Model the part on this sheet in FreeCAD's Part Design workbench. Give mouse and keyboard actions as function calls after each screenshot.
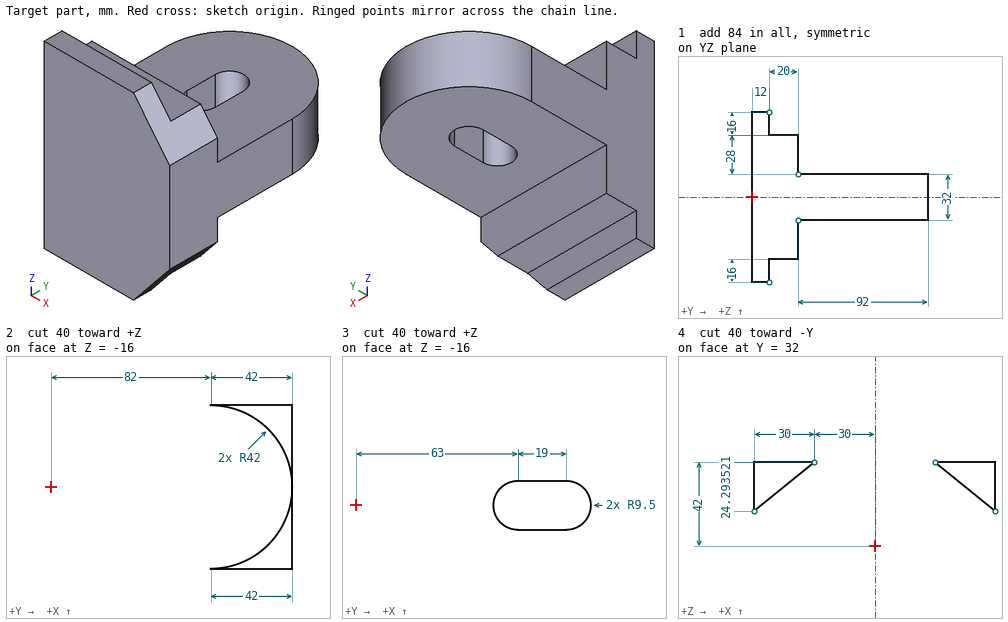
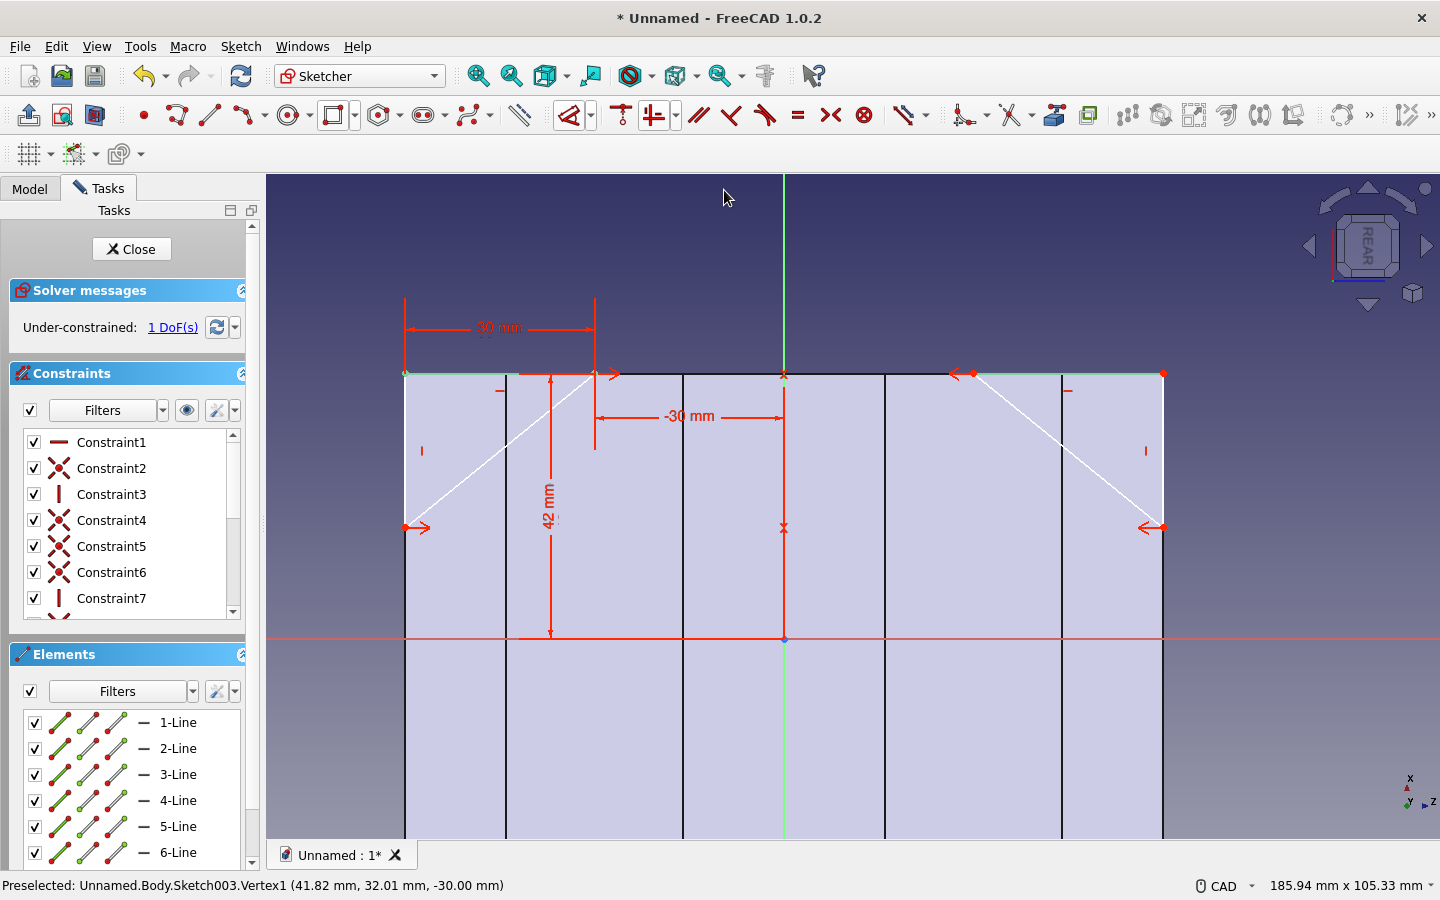
click(405, 420)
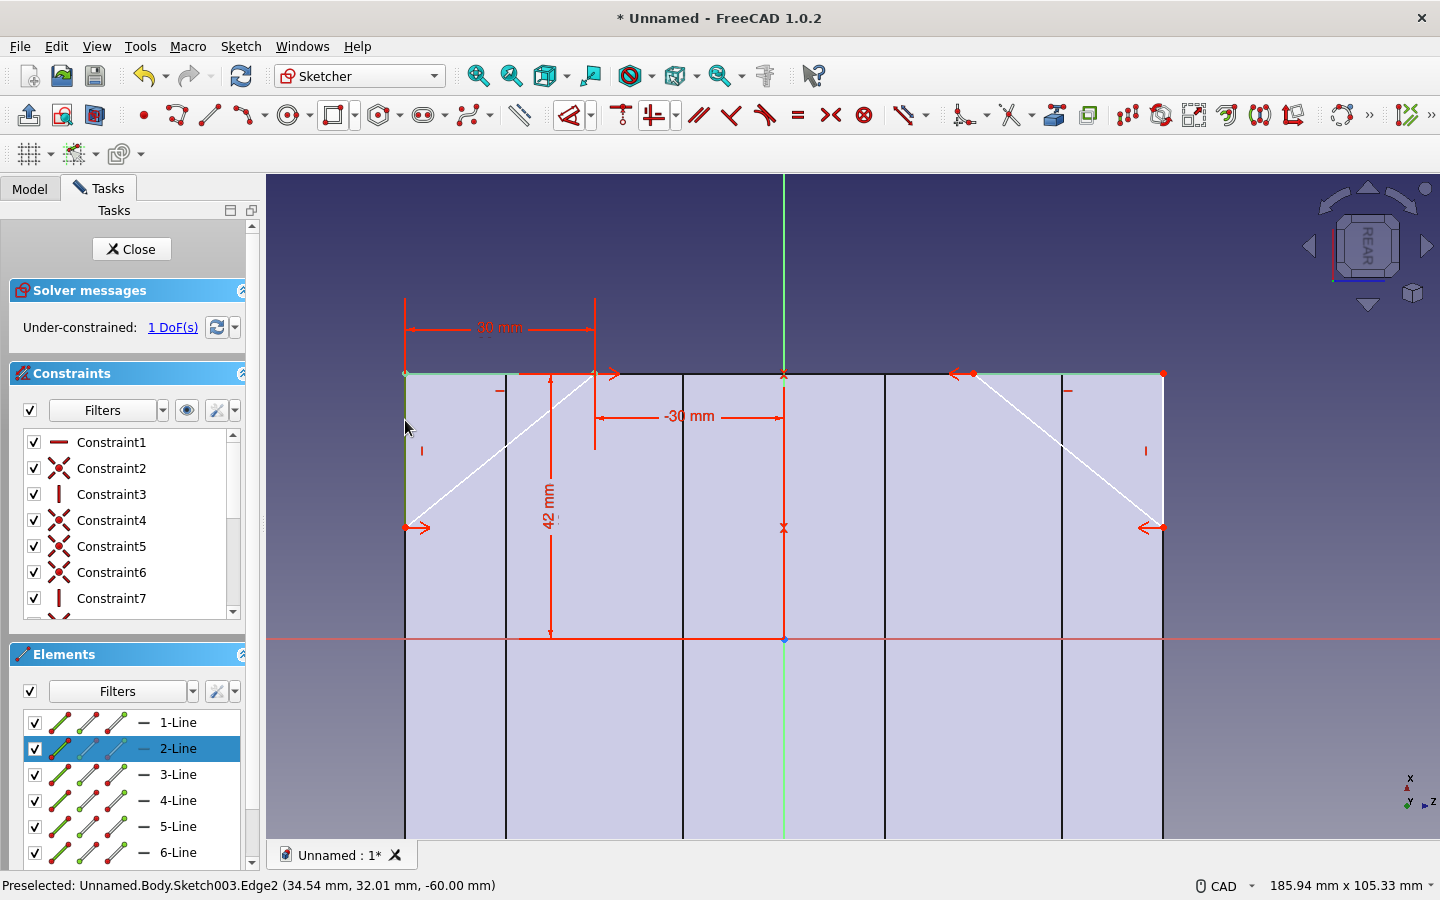
key(i)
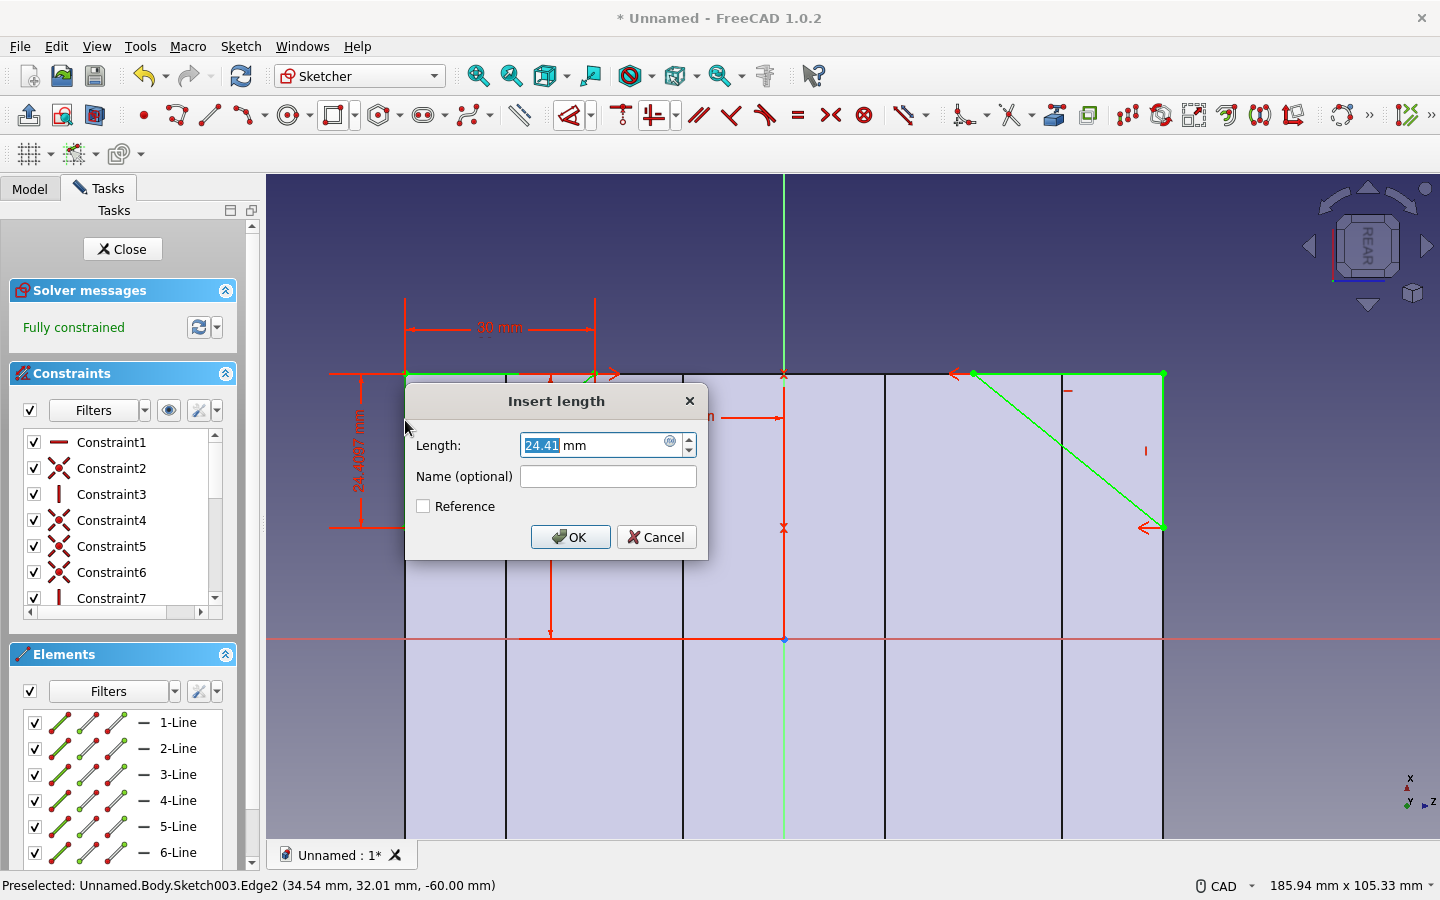
text(24.293521)
key(Return)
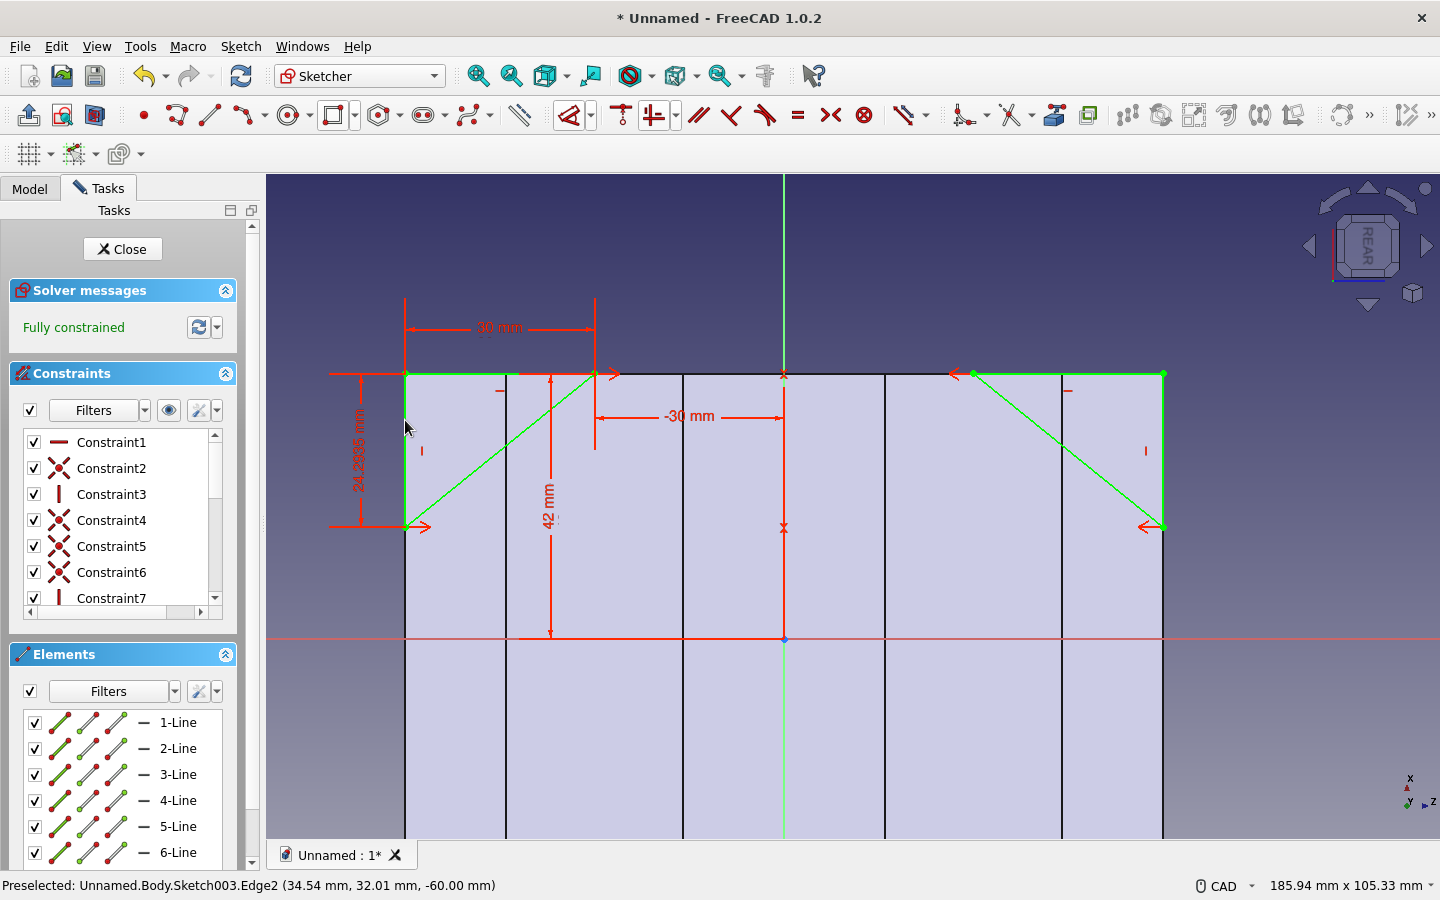
click(123, 249)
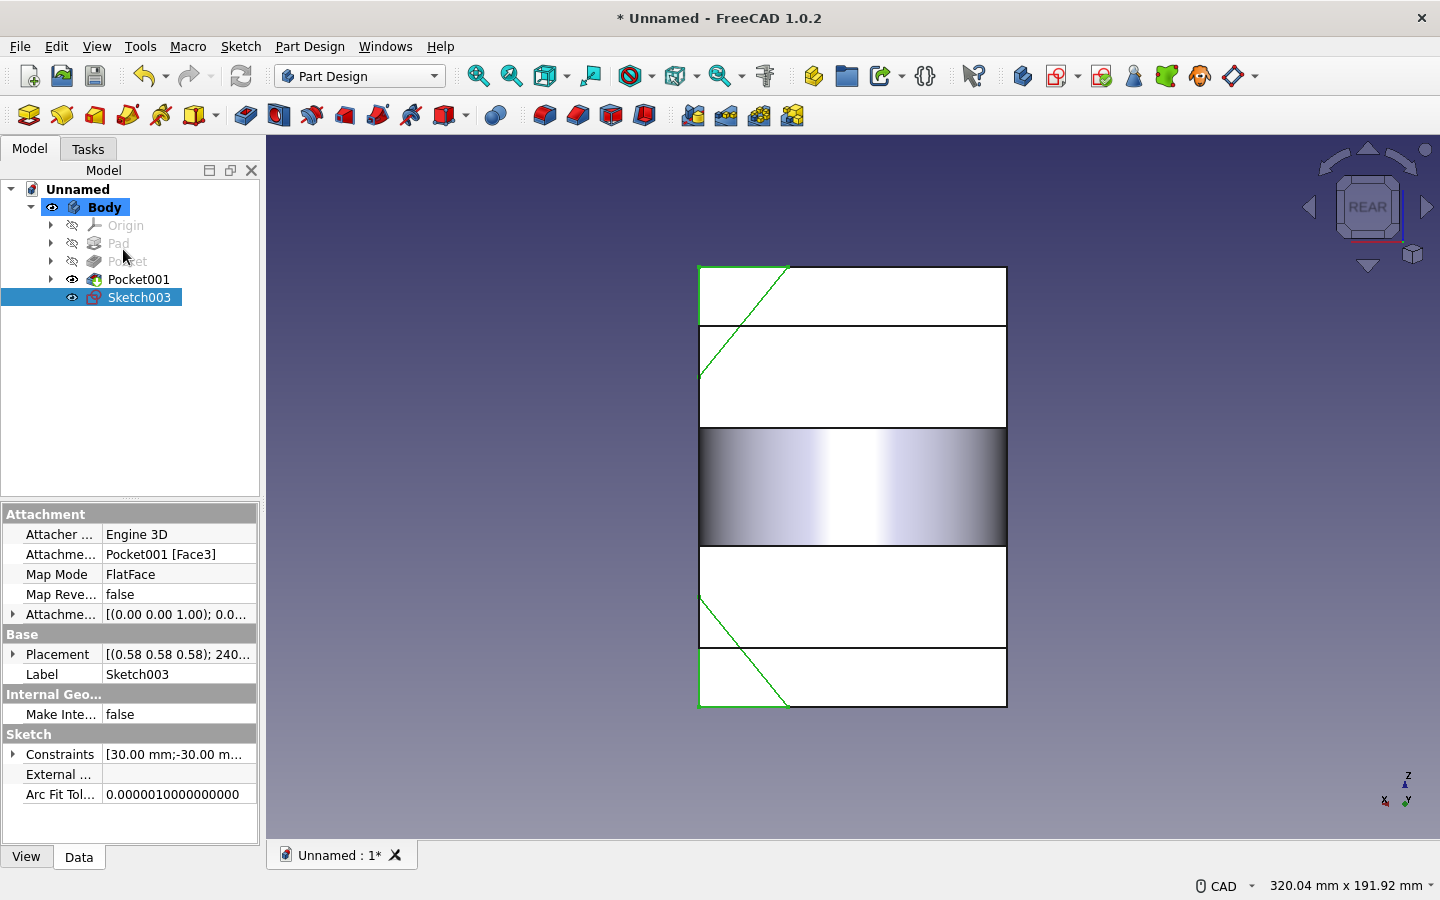
click(246, 116)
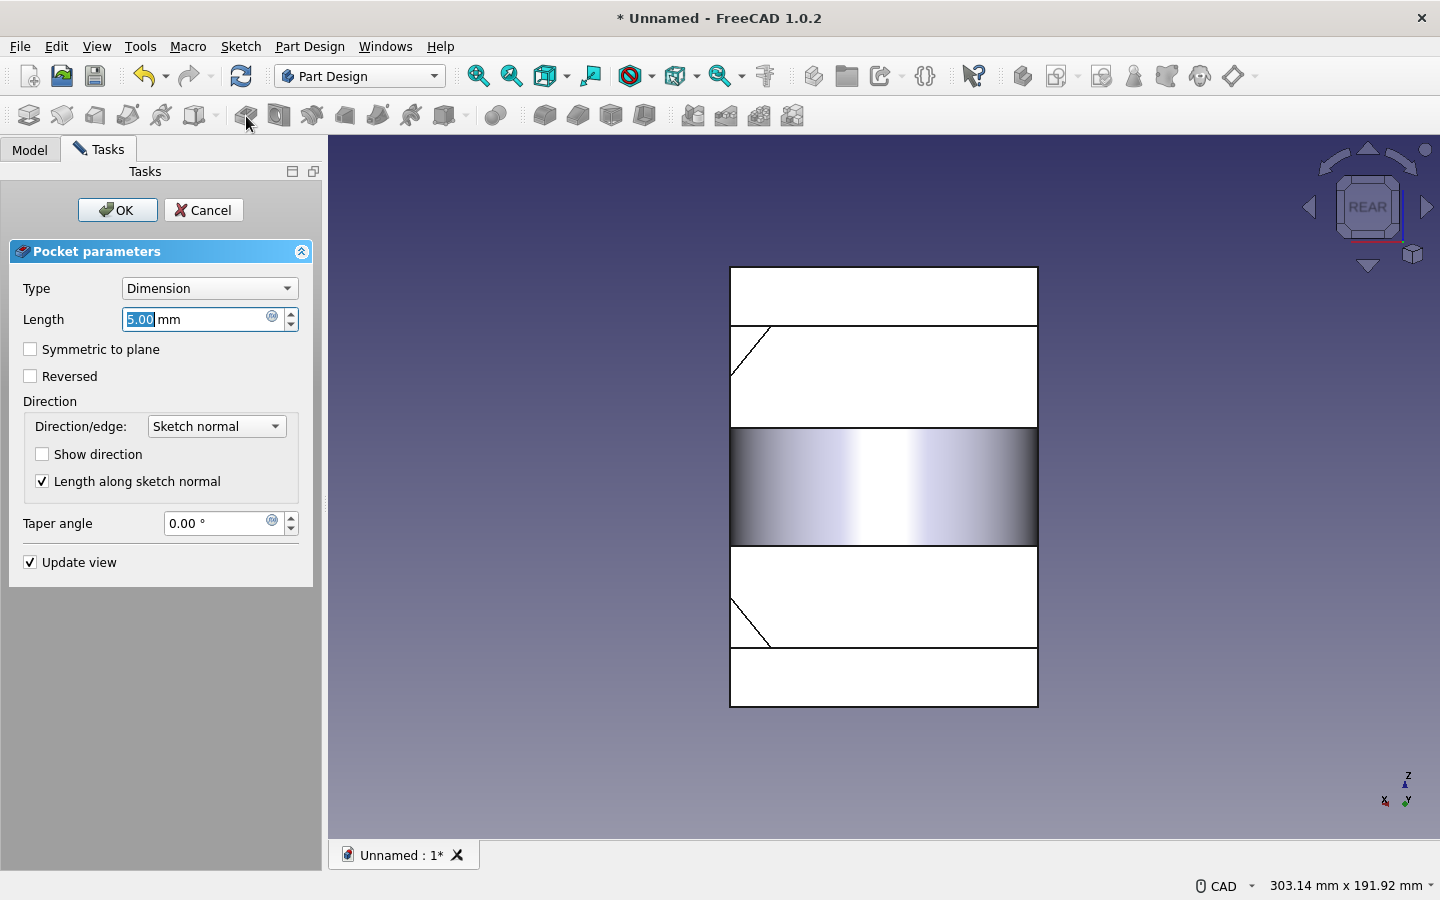
text(40)
key(Tab)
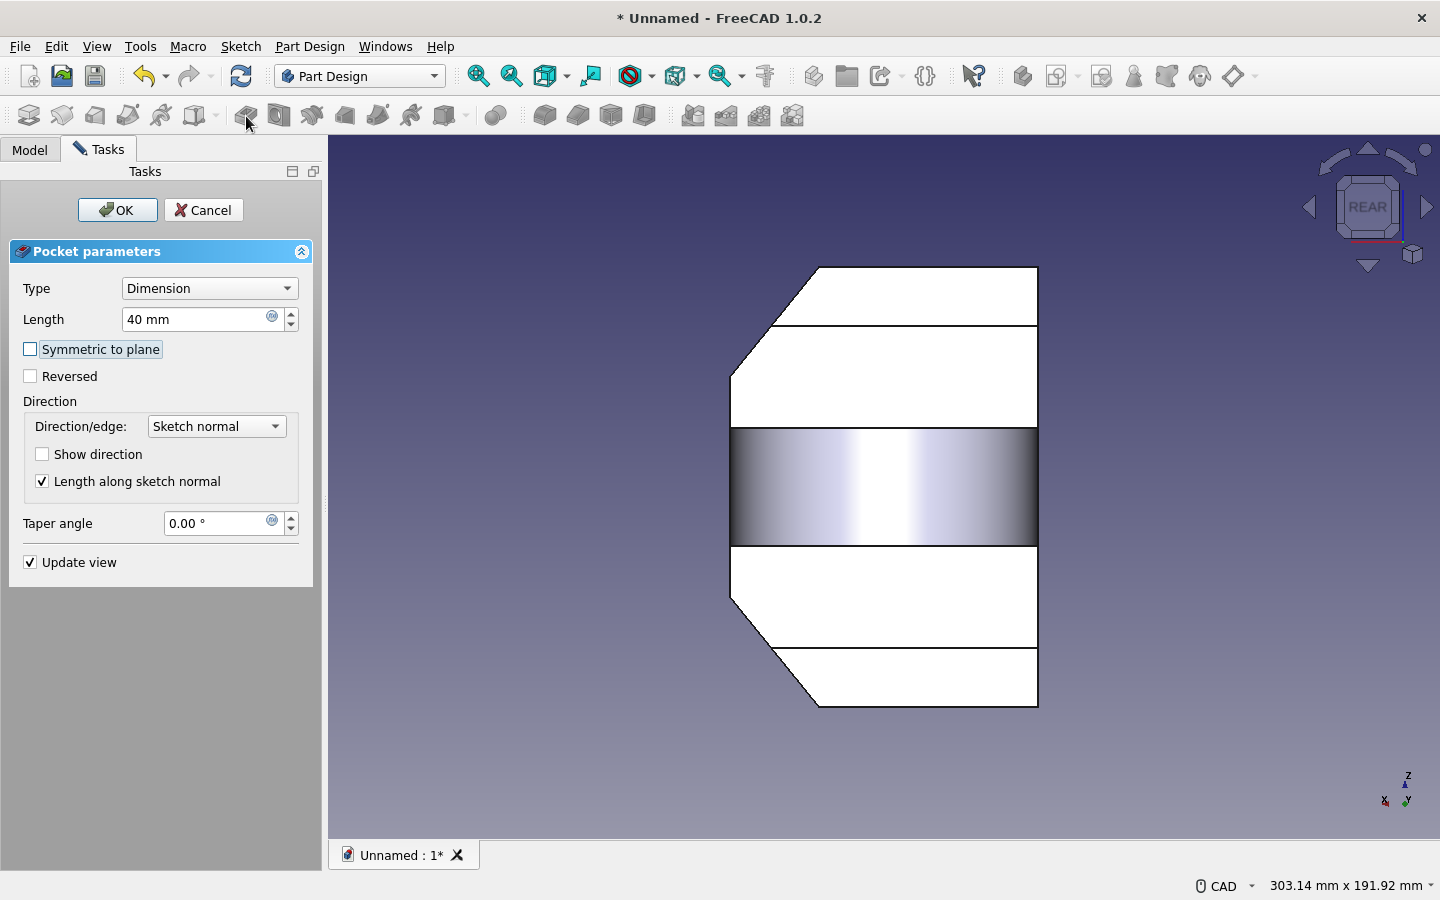
click(118, 210)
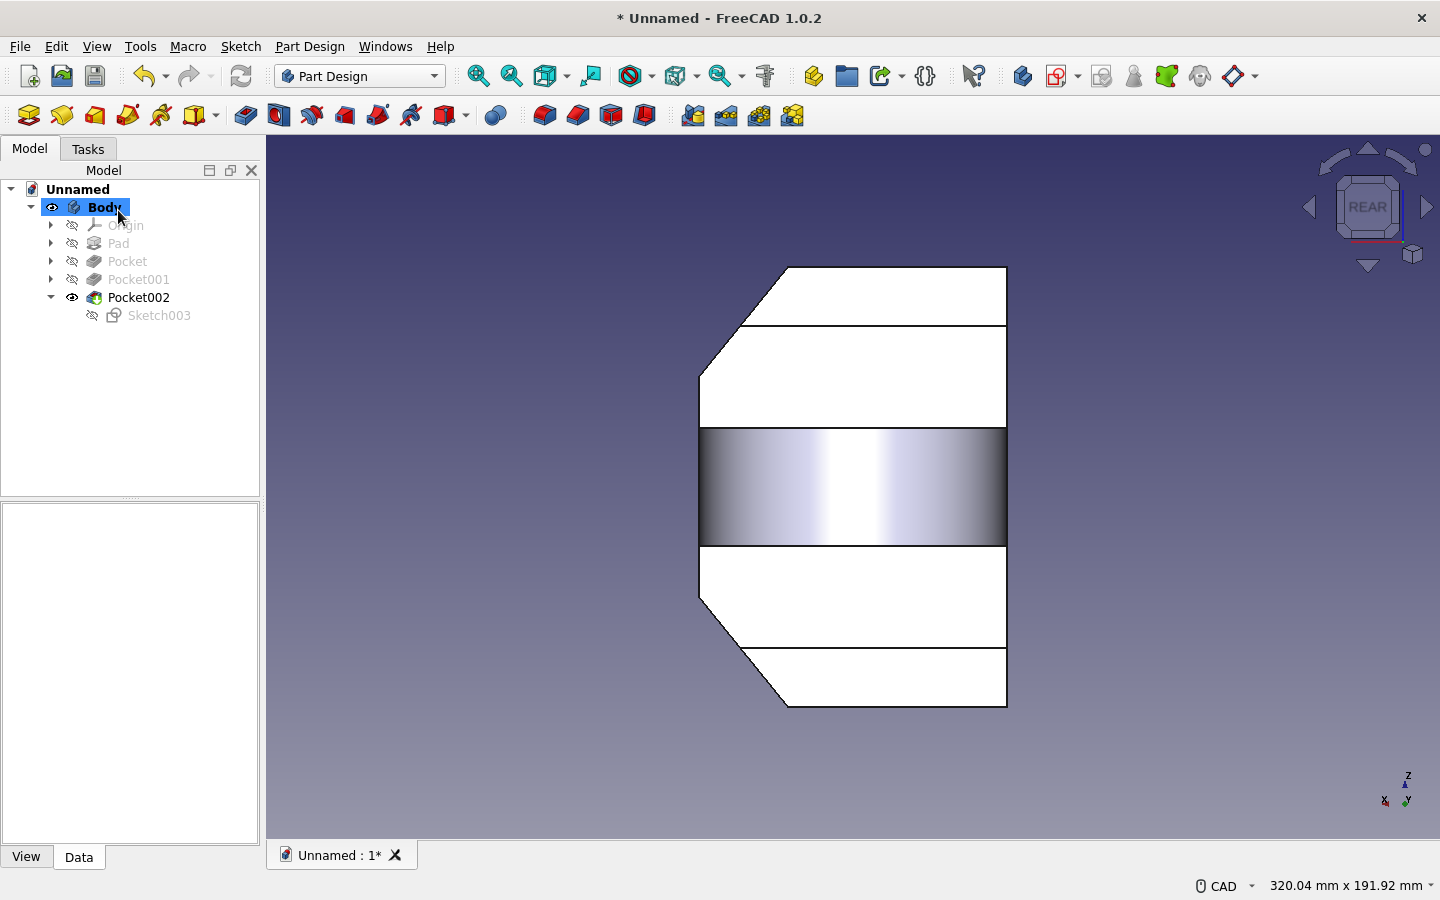
key(0)